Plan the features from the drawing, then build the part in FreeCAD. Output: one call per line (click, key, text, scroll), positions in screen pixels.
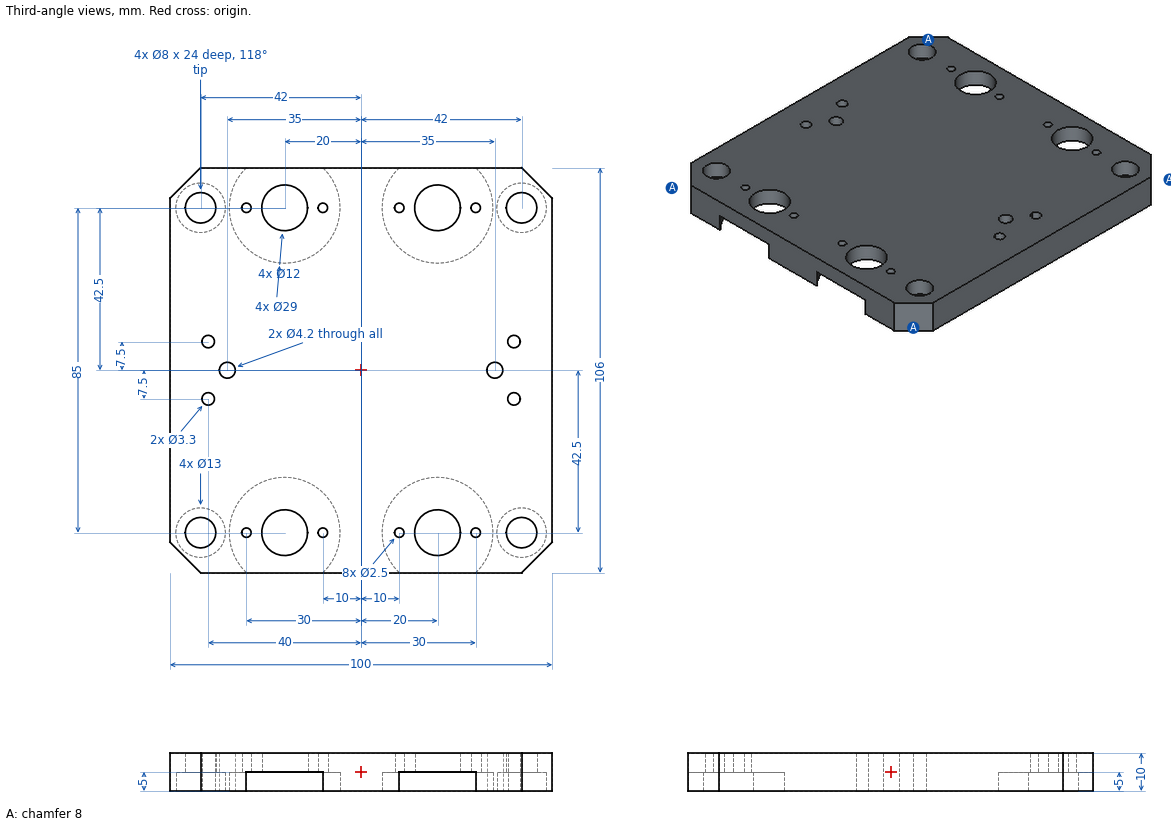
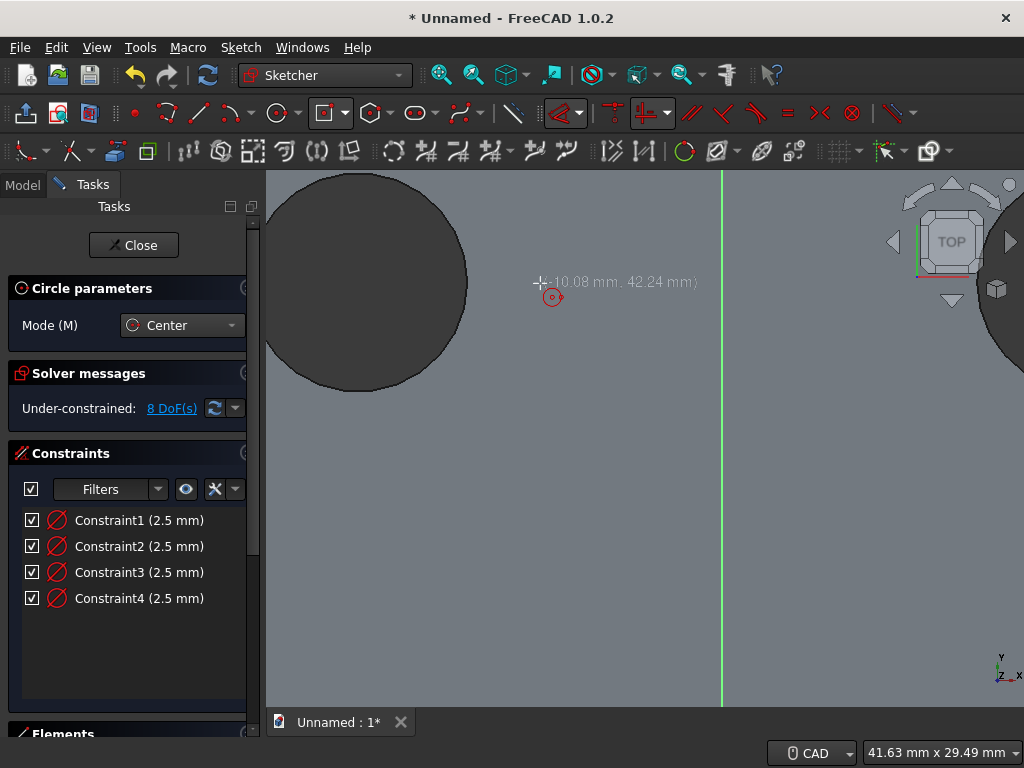
scroll(540, 282, down, 8)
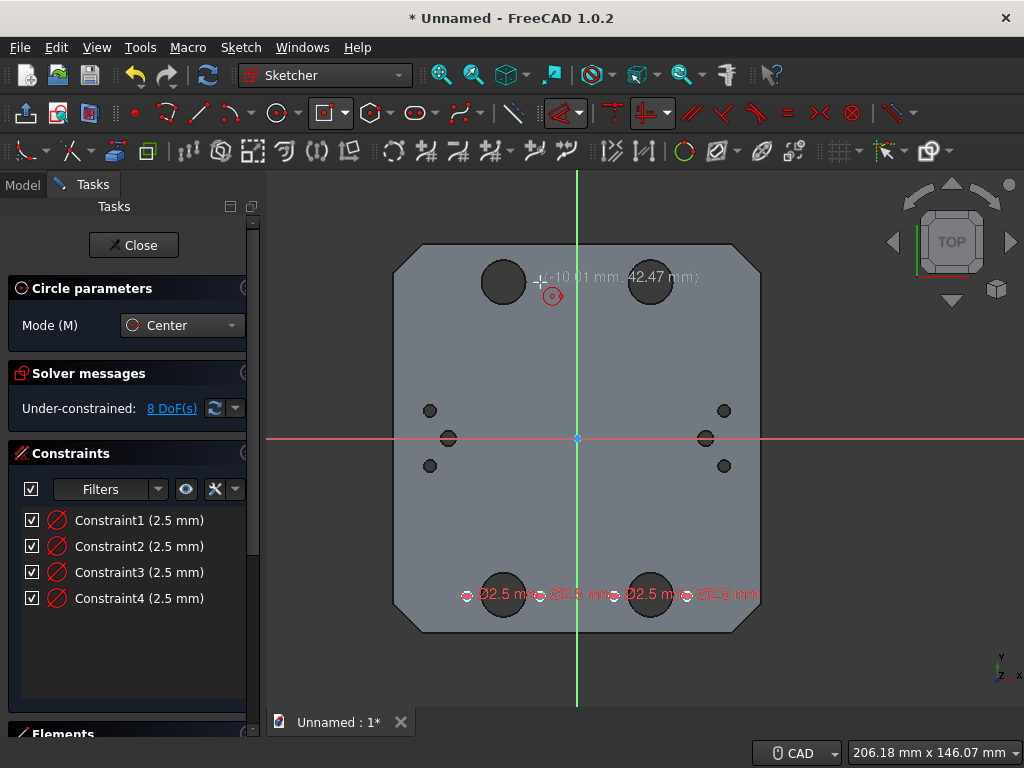
click(540, 282)
move(544, 279)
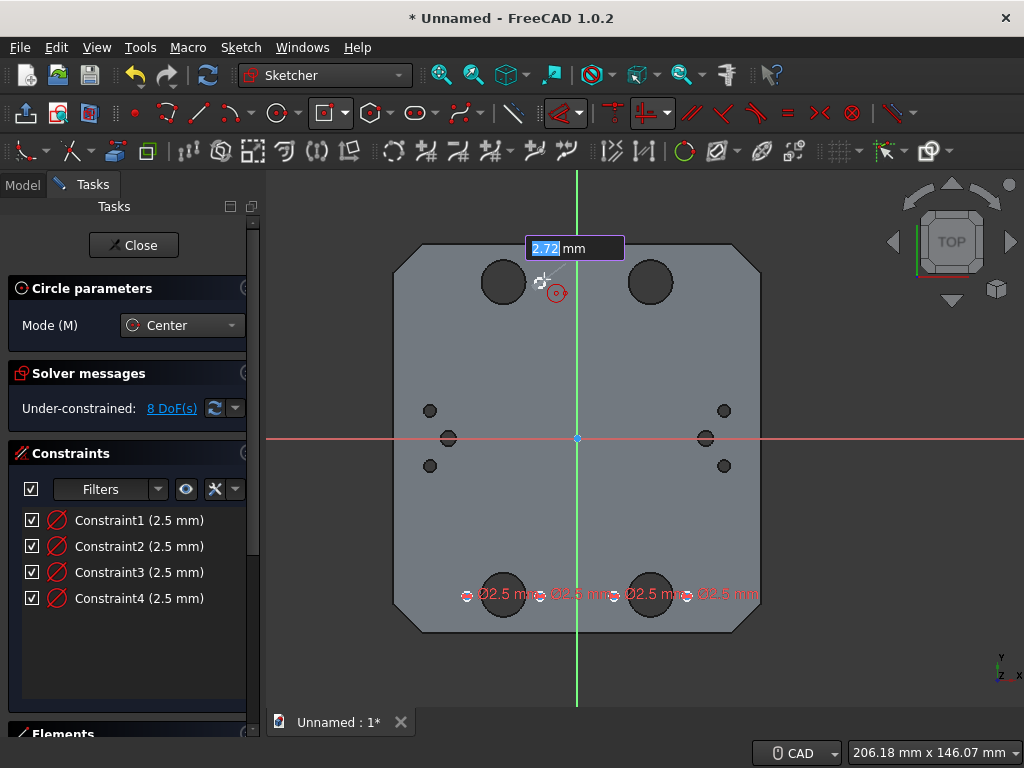
text(2.5)
key(Return)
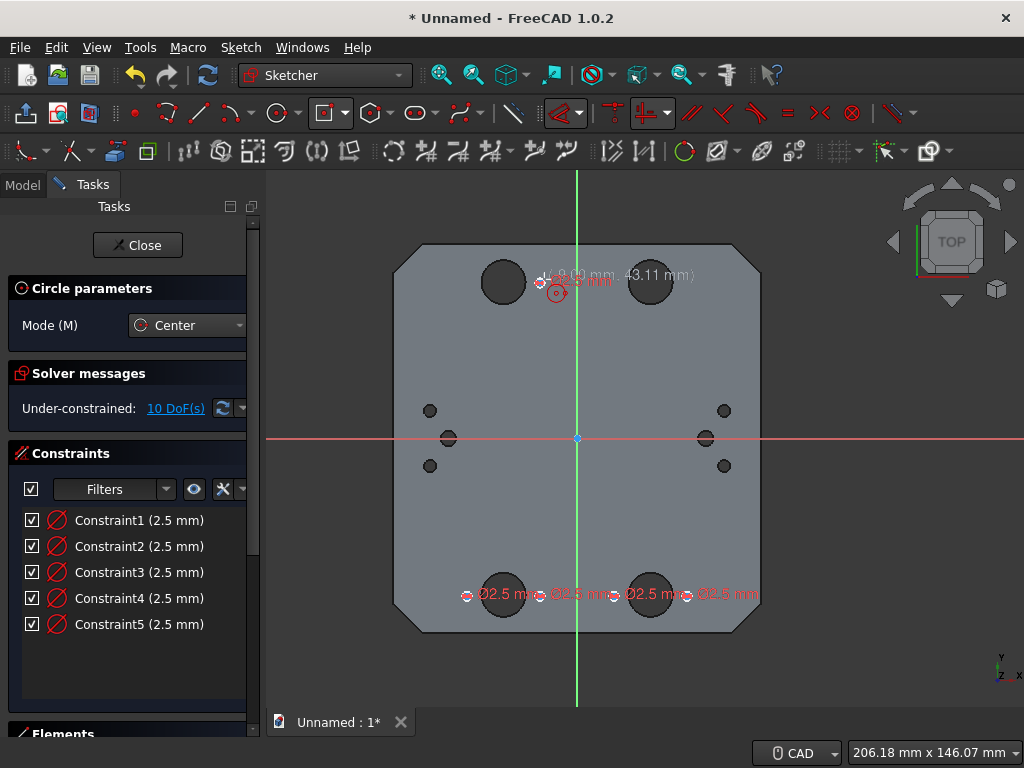
scroll(467, 282, up, 8)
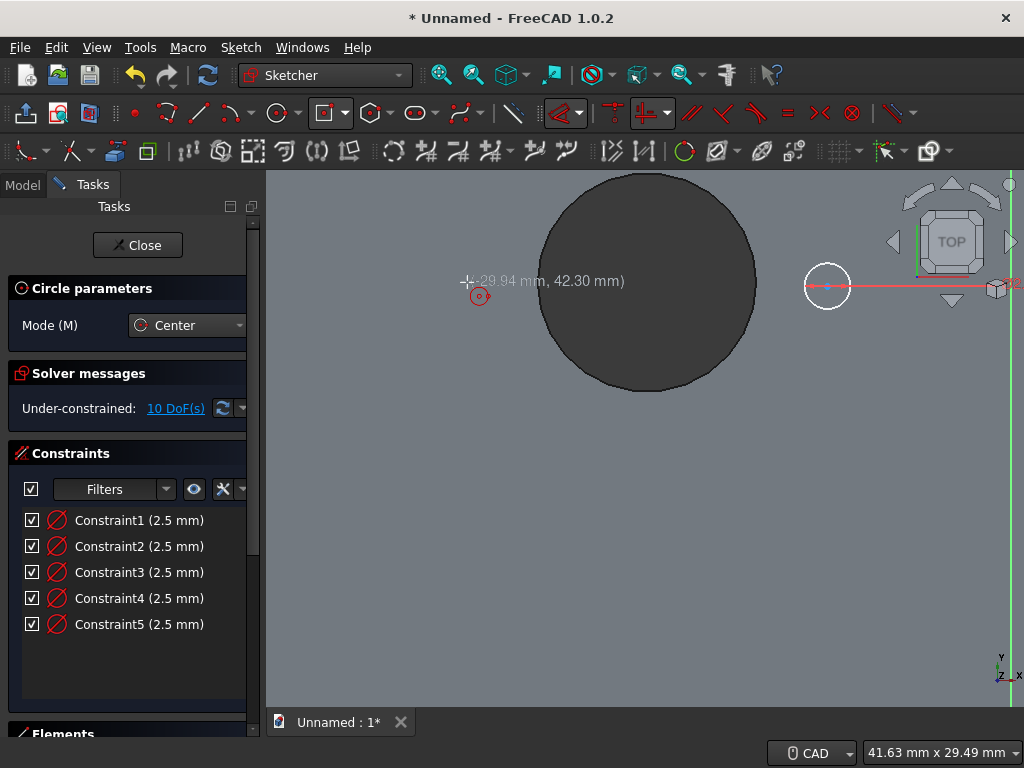
scroll(467, 282, down, 8)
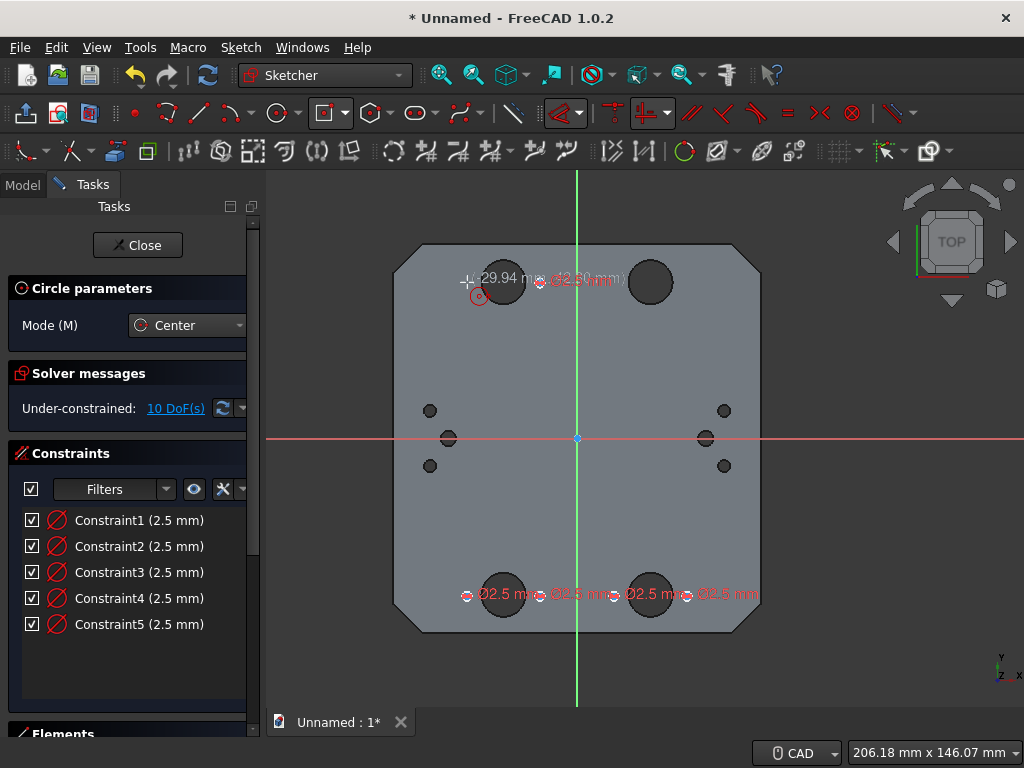
click(467, 282)
move(470, 279)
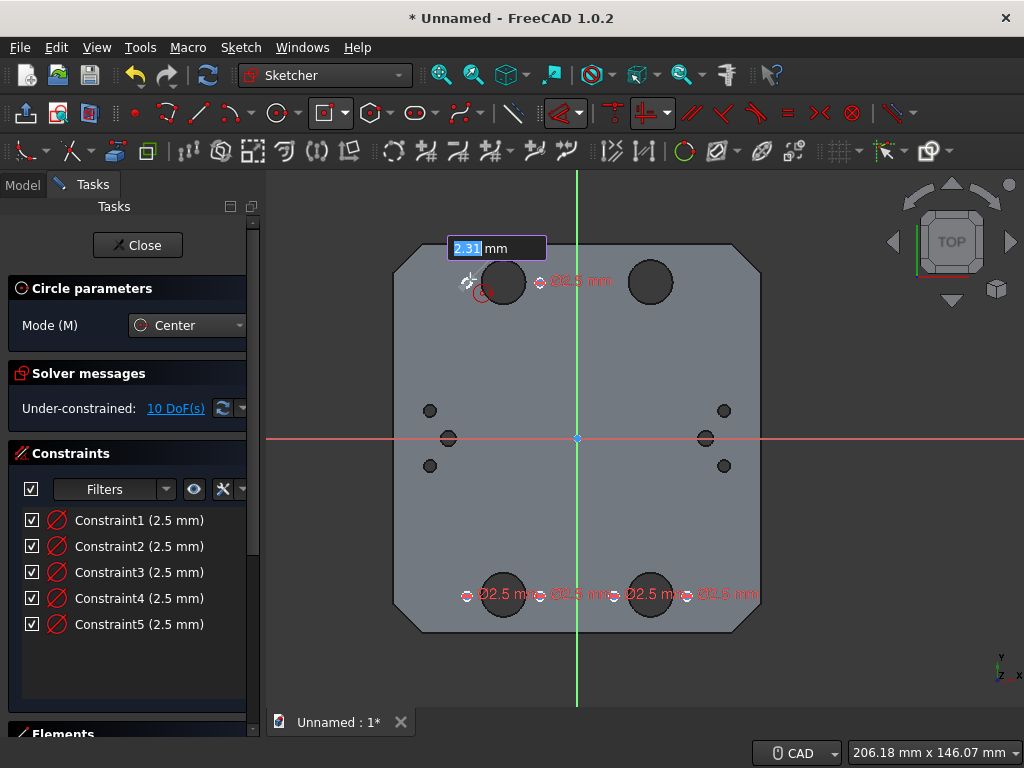
text(2.5)
key(Return)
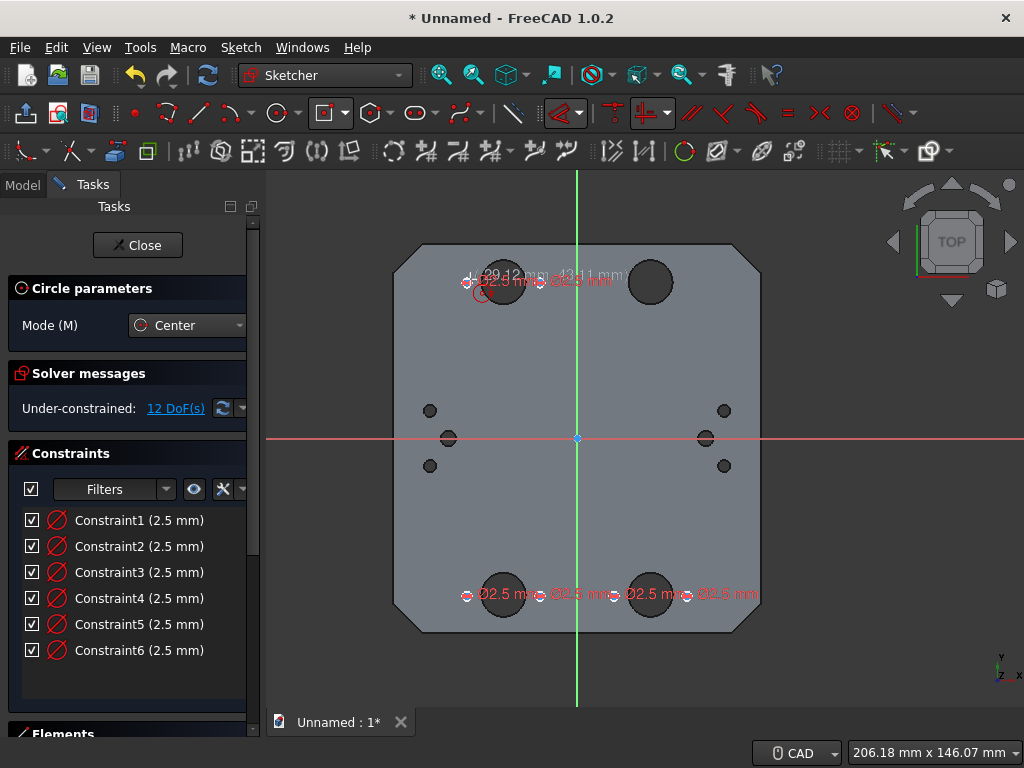
scroll(614, 282, up, 8)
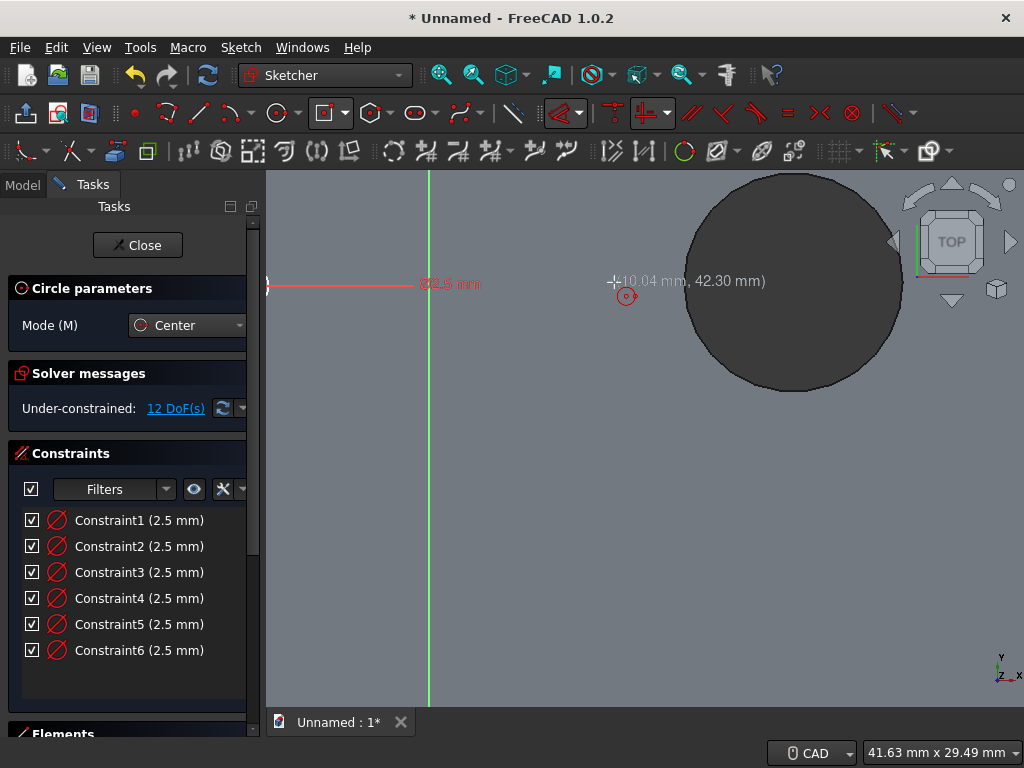
scroll(614, 282, down, 8)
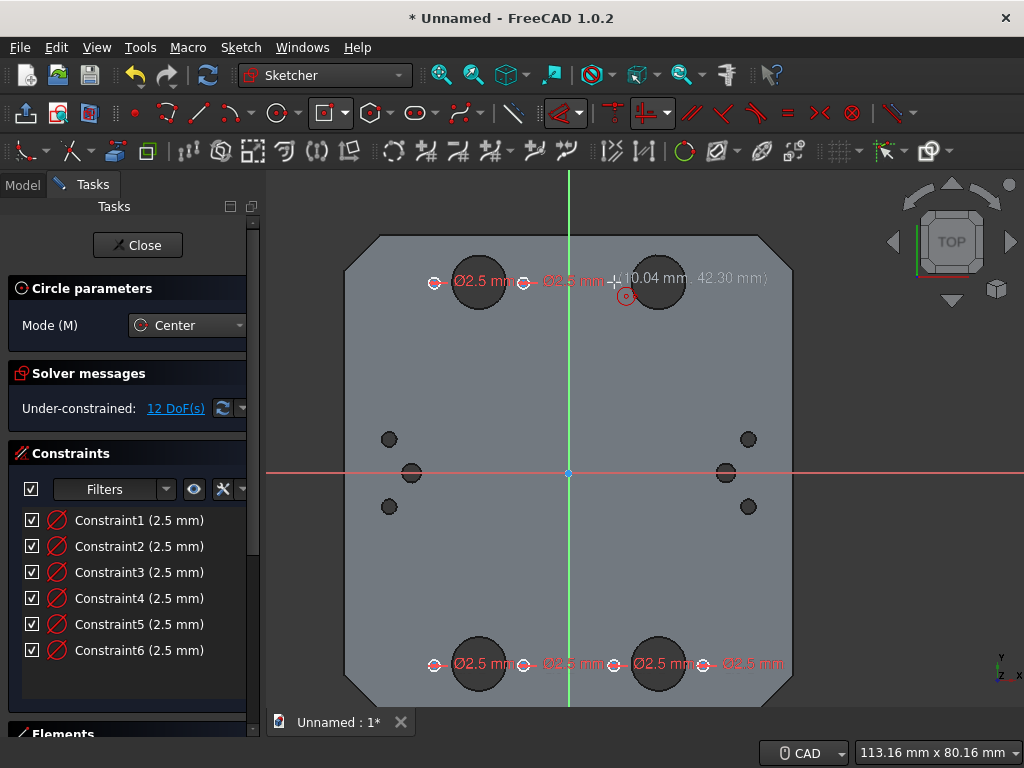
click(614, 282)
move(617, 279)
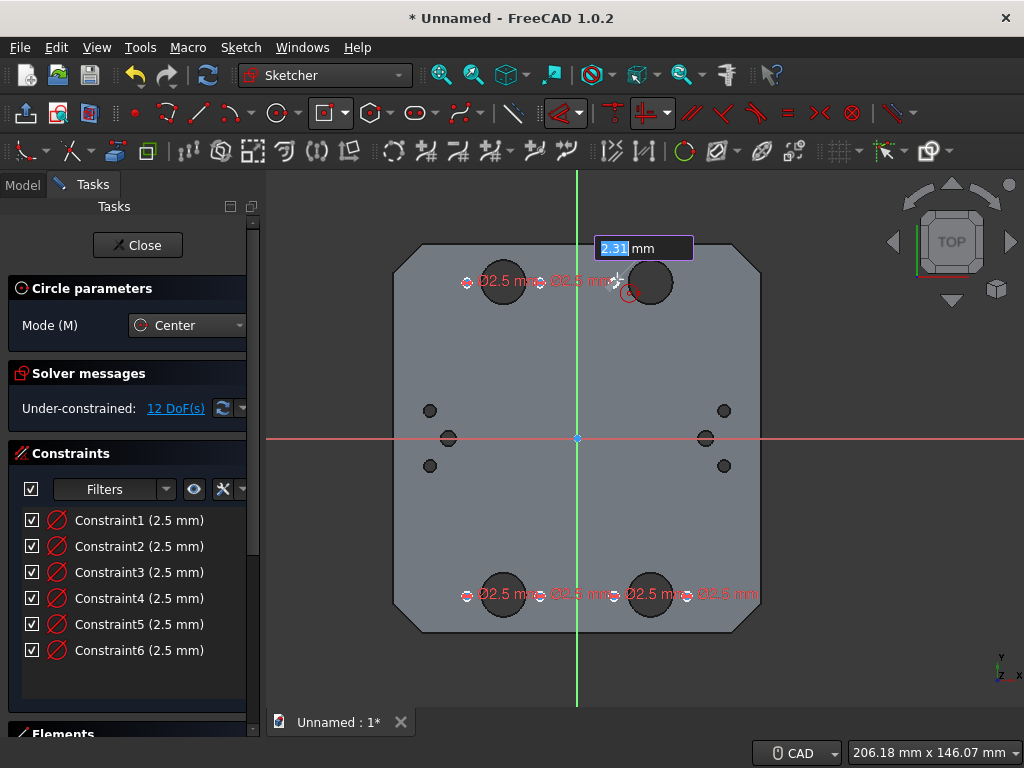
text(2.5)
key(Return)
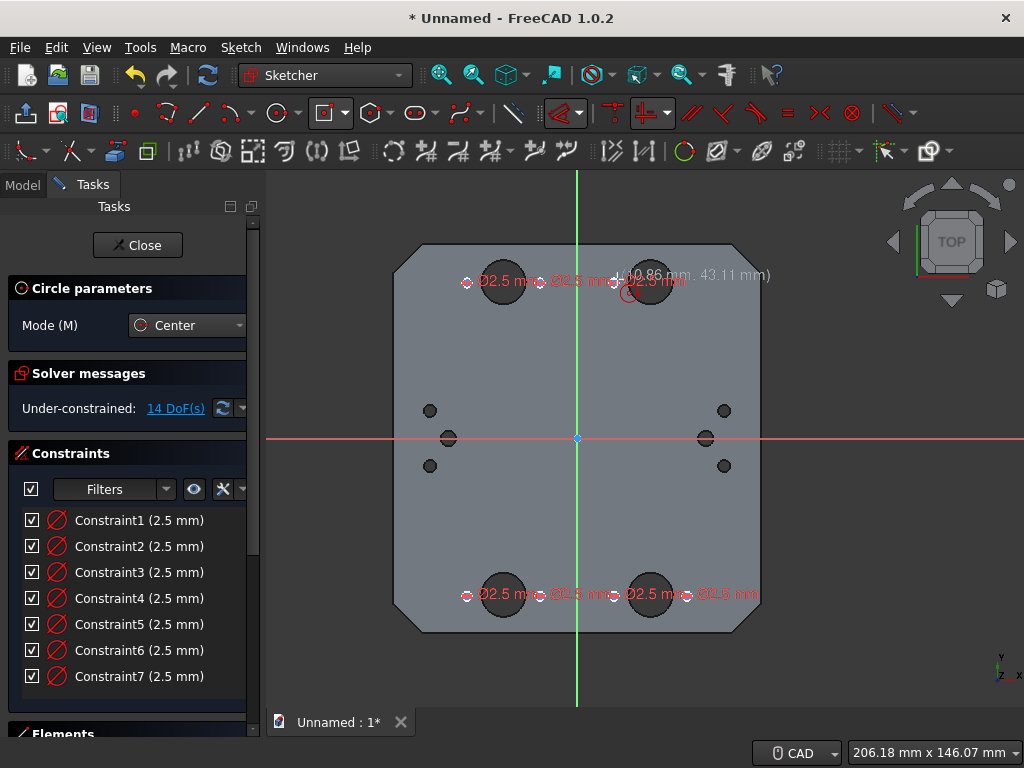
scroll(687, 282, up, 8)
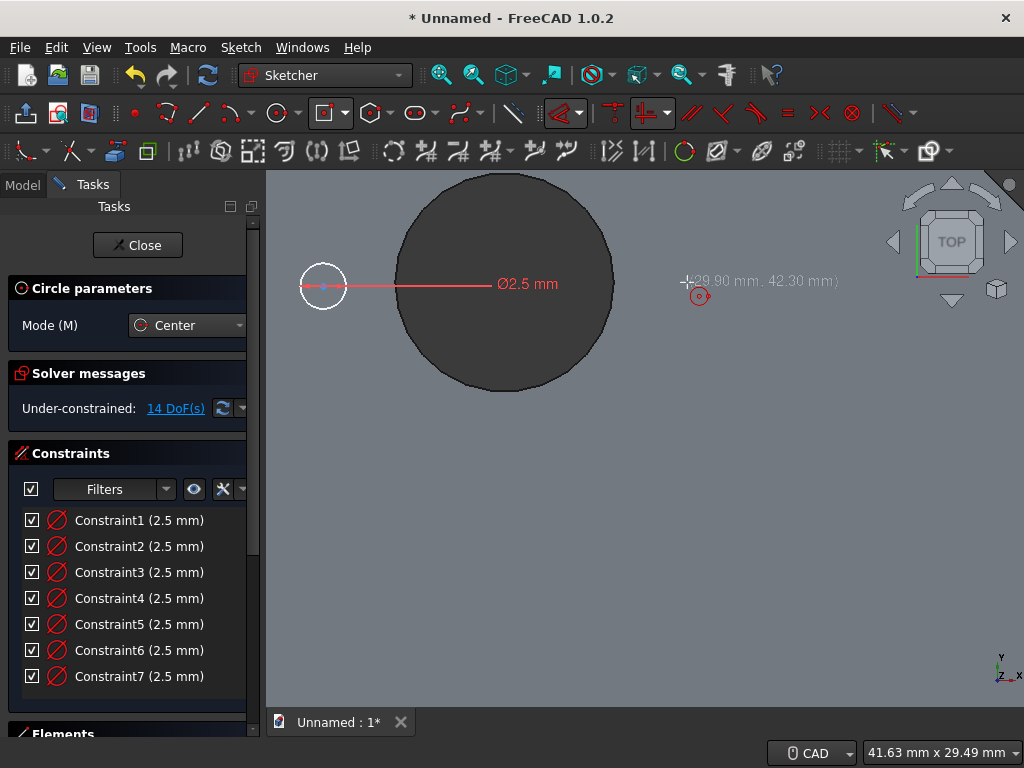
scroll(687, 282, down, 8)